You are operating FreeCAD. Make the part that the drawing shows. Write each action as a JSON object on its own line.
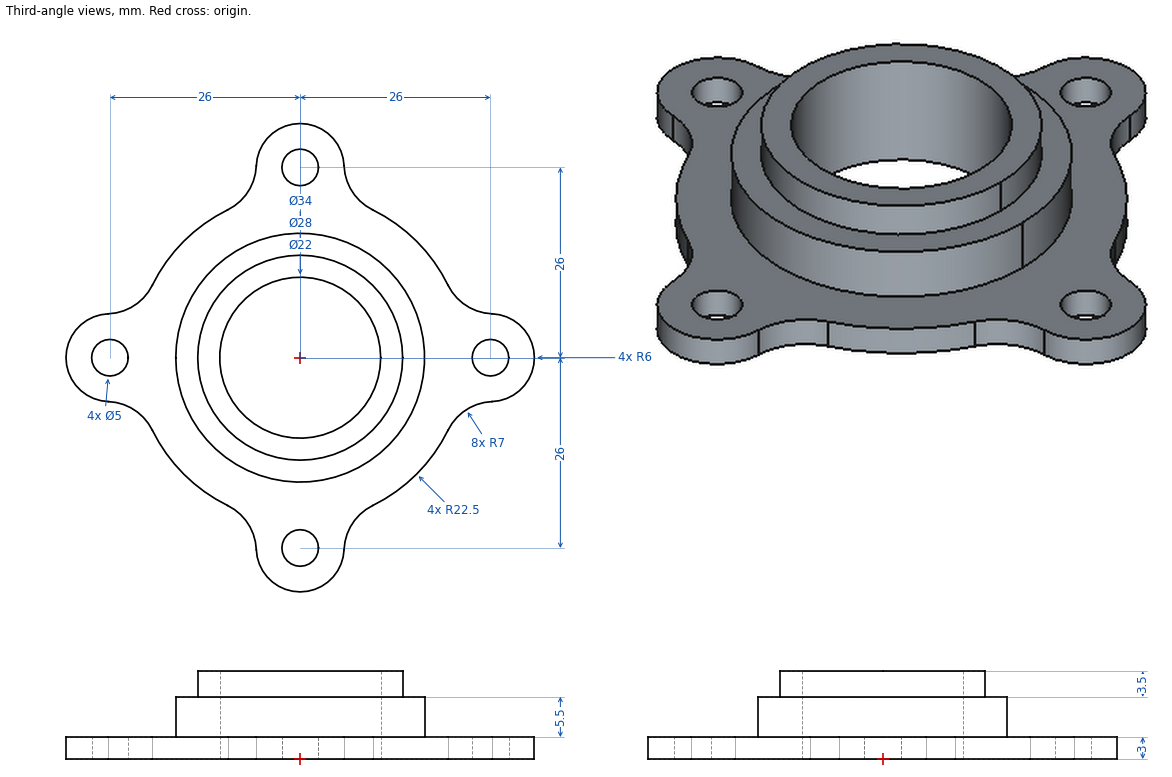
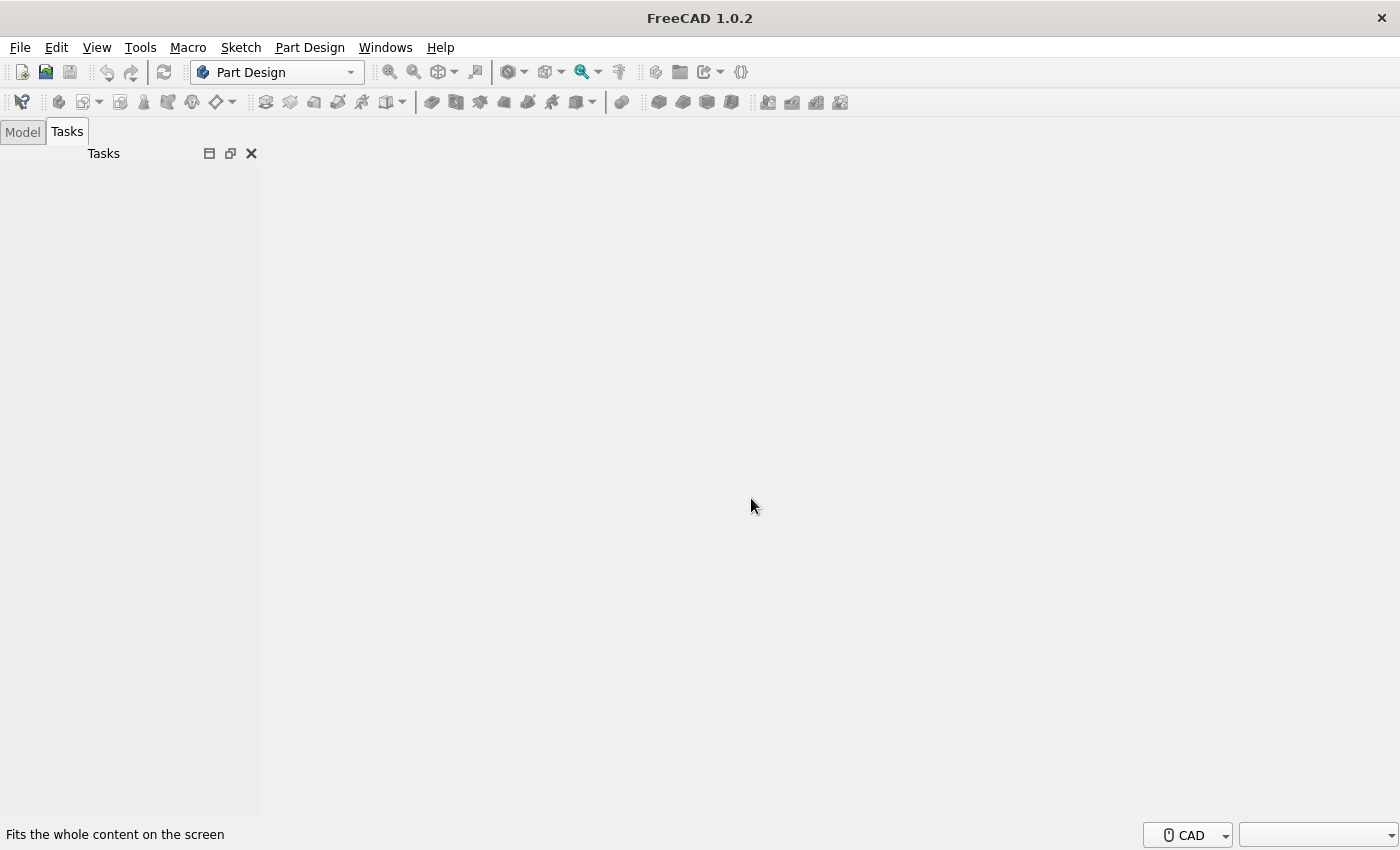
{"action": "left_click", "coordinate": [22, 72]}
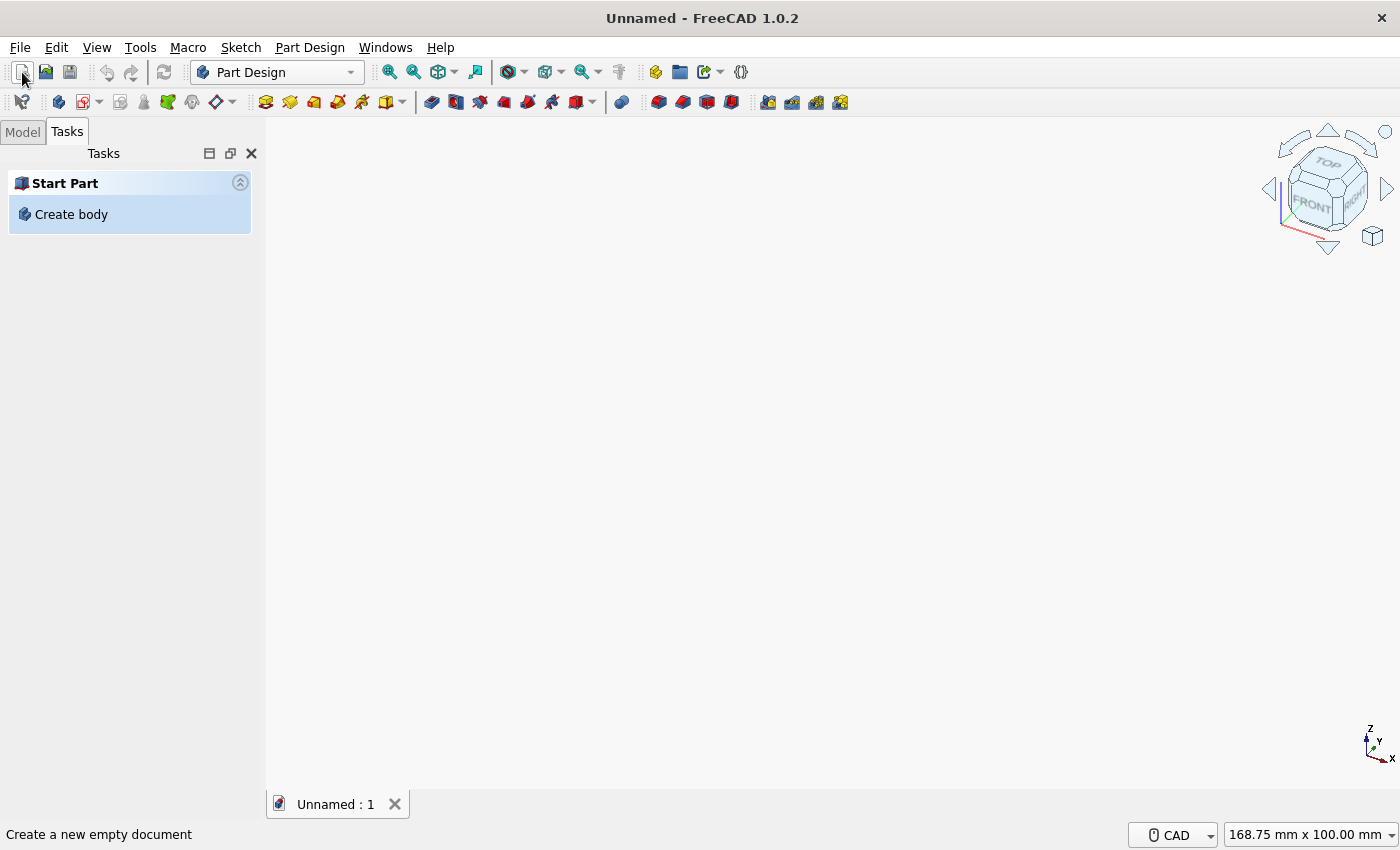
{"action": "left_click", "coordinate": [84, 102]}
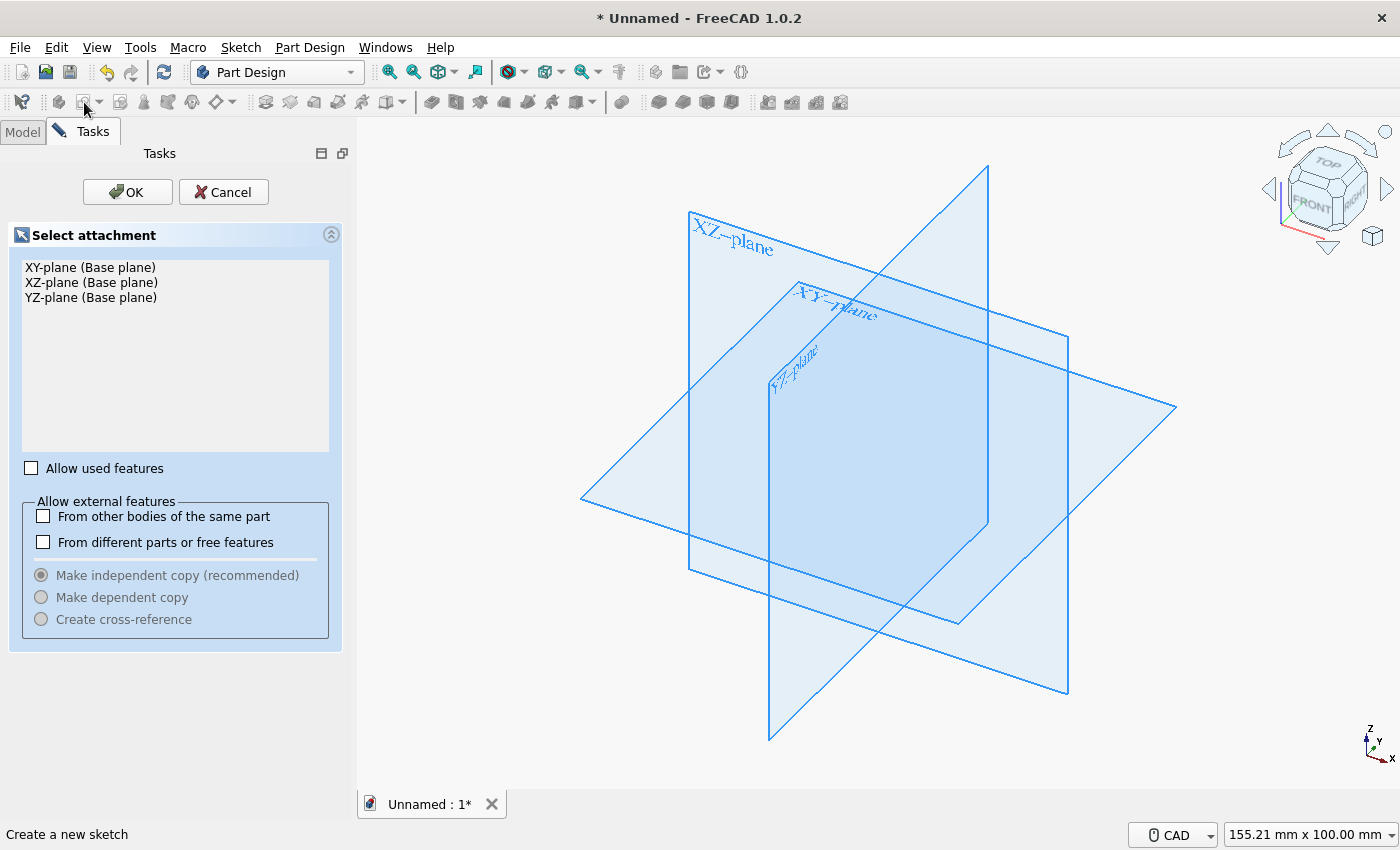
{"action": "left_click", "coordinate": [82, 268]}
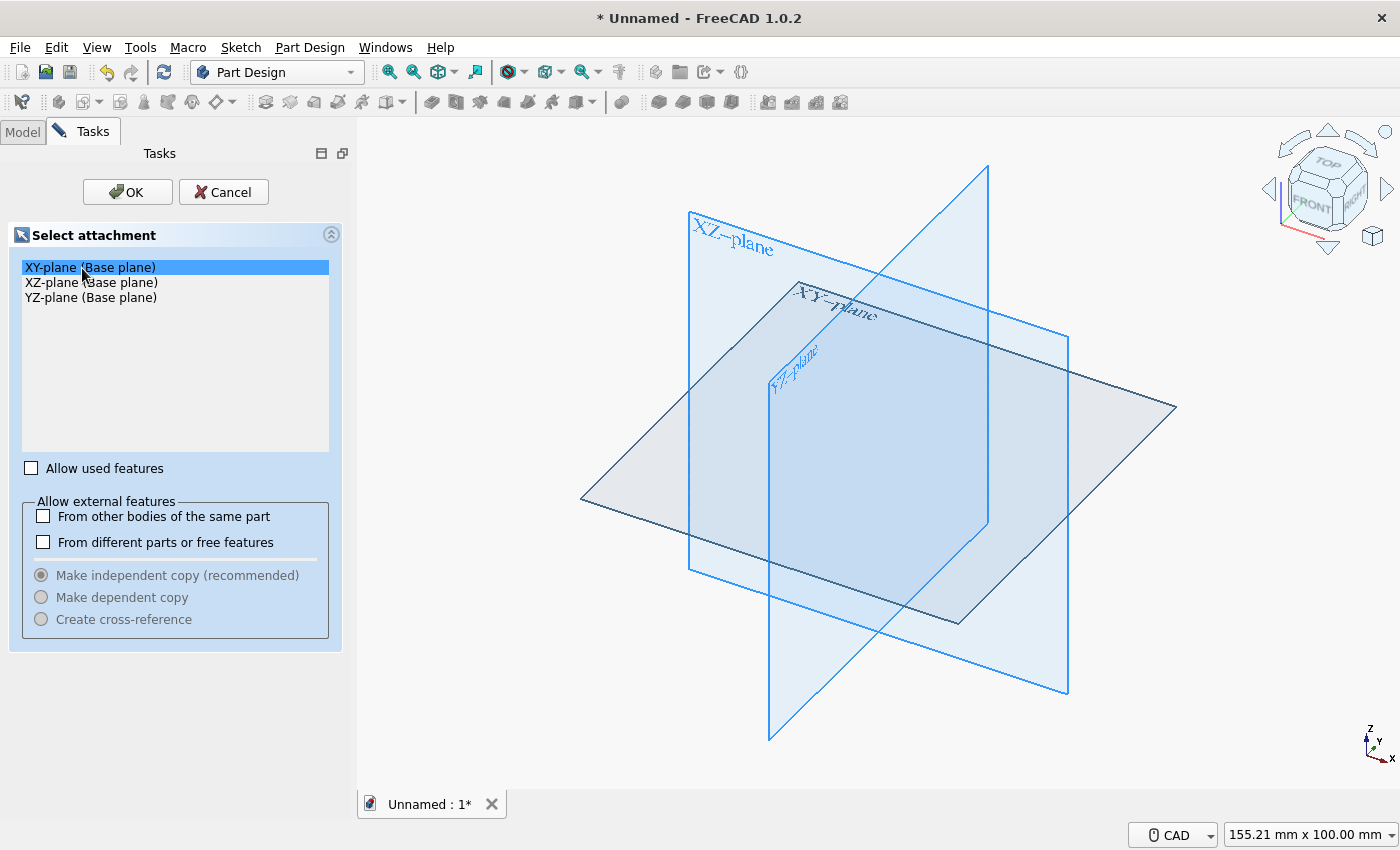
{"action": "left_click", "coordinate": [128, 192]}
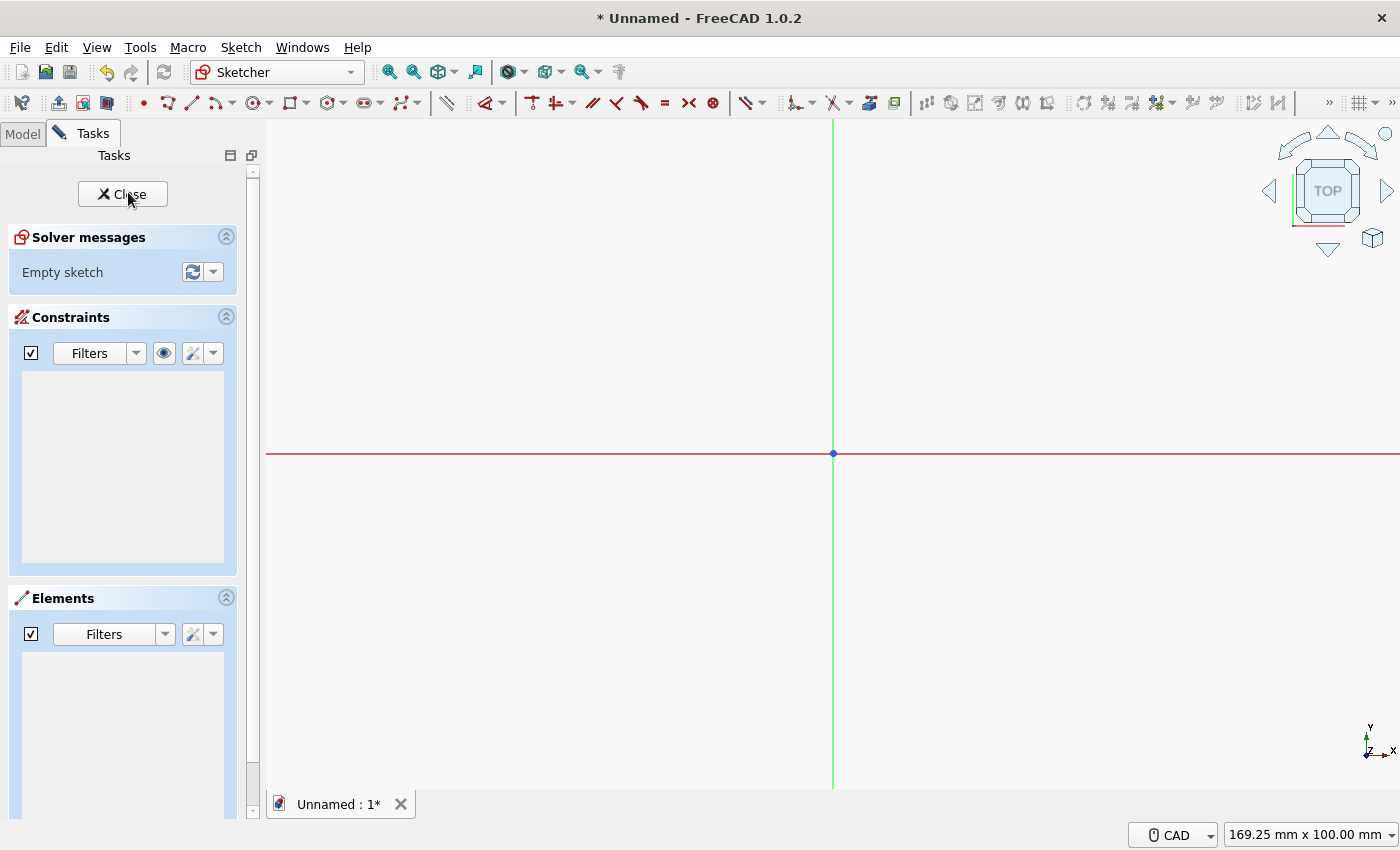
{"action": "key", "text": "g 3 a"}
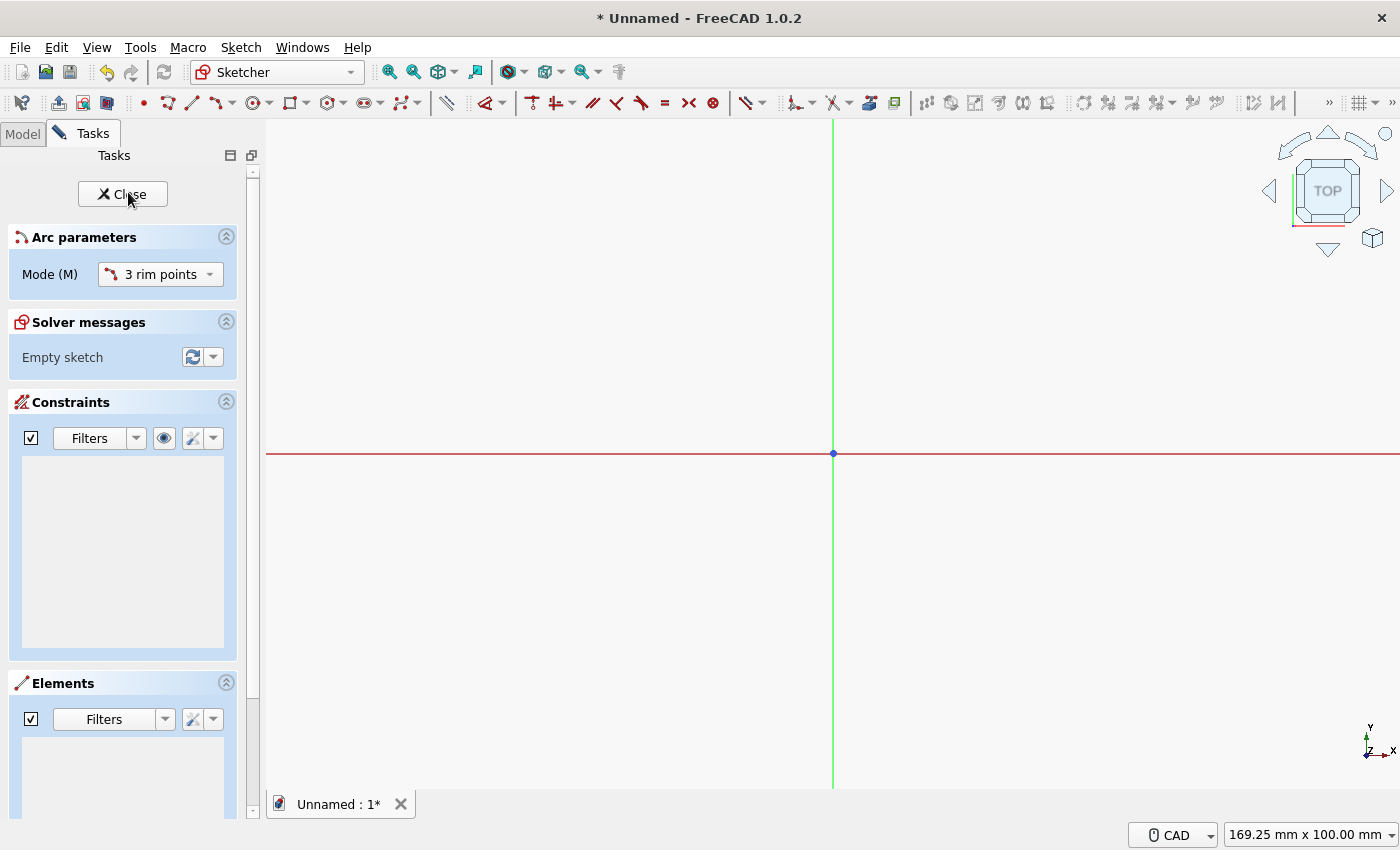
{"action": "left_click", "coordinate": [899, 589]}
{"action": "left_click", "coordinate": [968, 520]}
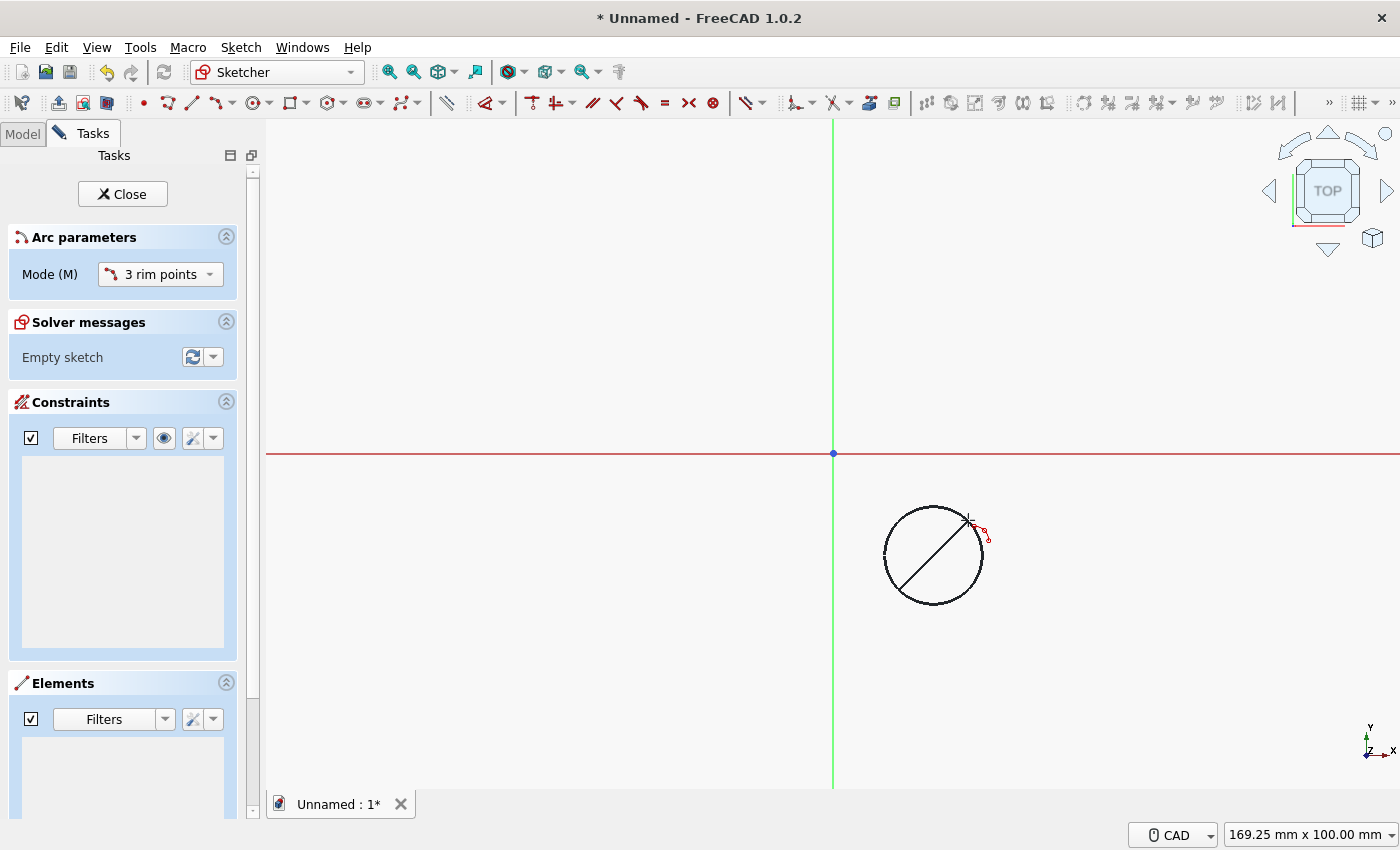
{"action": "scroll", "coordinate": [940, 561], "scroll_direction": "up", "scroll_amount": 4}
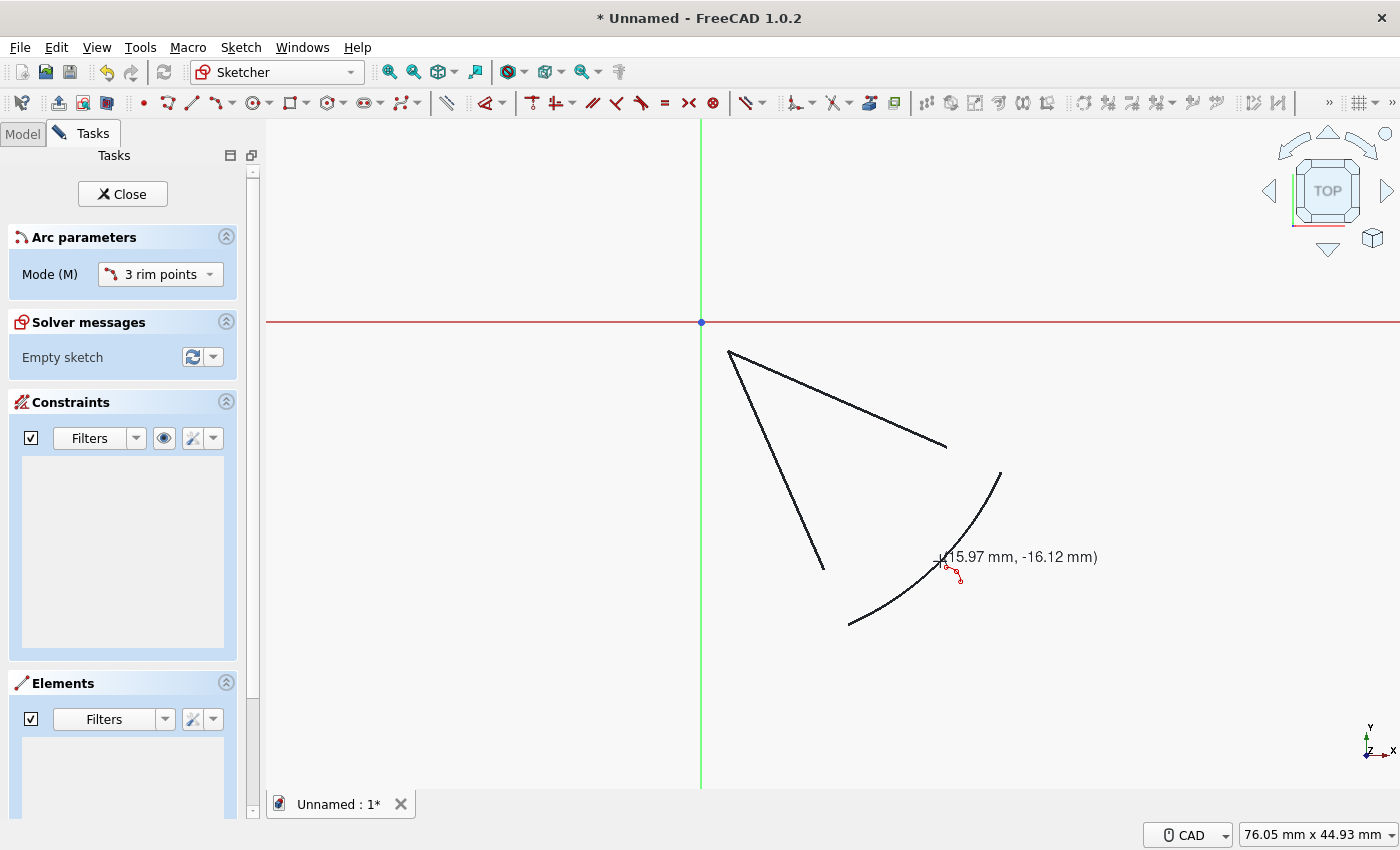
{"action": "left_click", "coordinate": [938, 559]}